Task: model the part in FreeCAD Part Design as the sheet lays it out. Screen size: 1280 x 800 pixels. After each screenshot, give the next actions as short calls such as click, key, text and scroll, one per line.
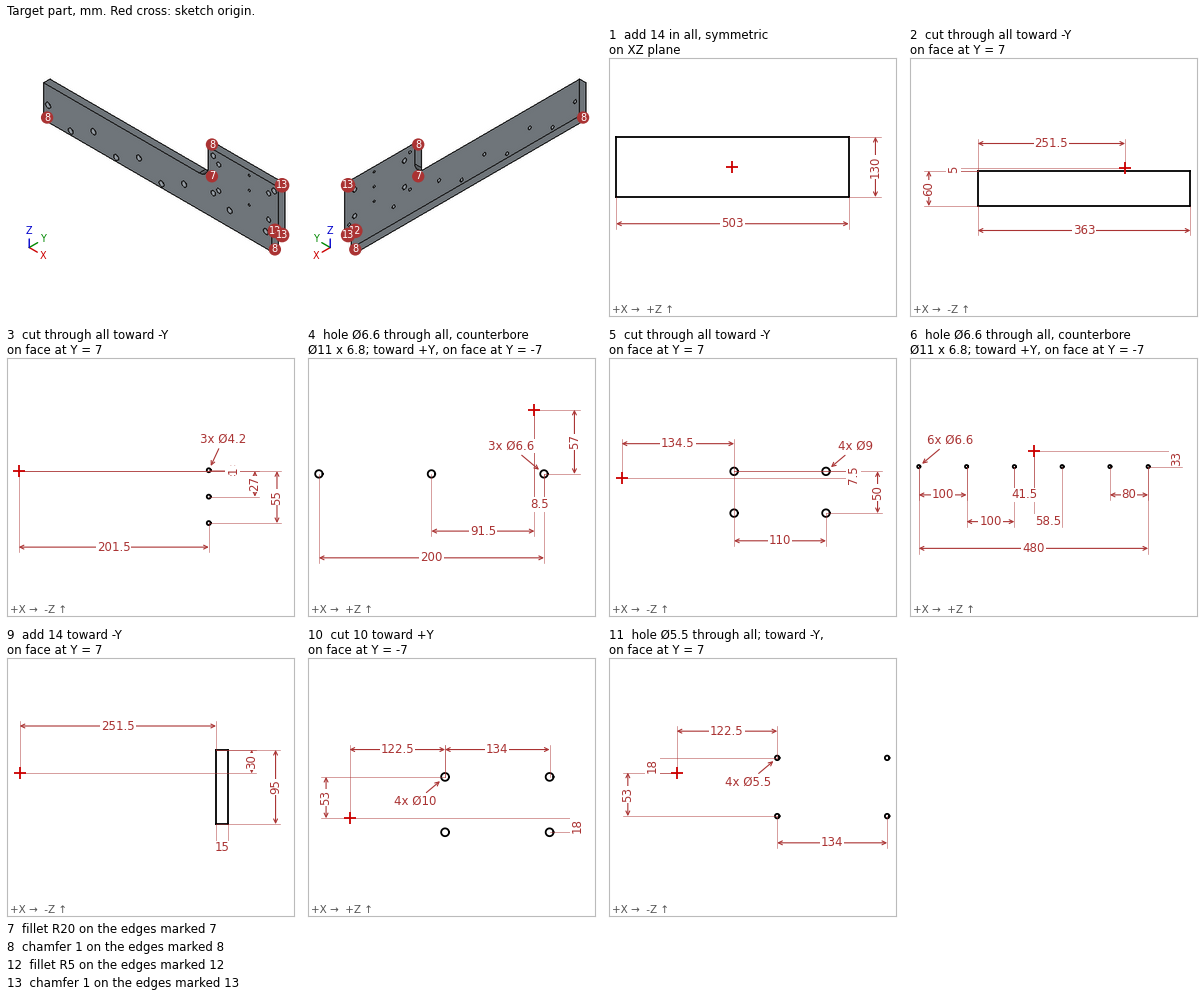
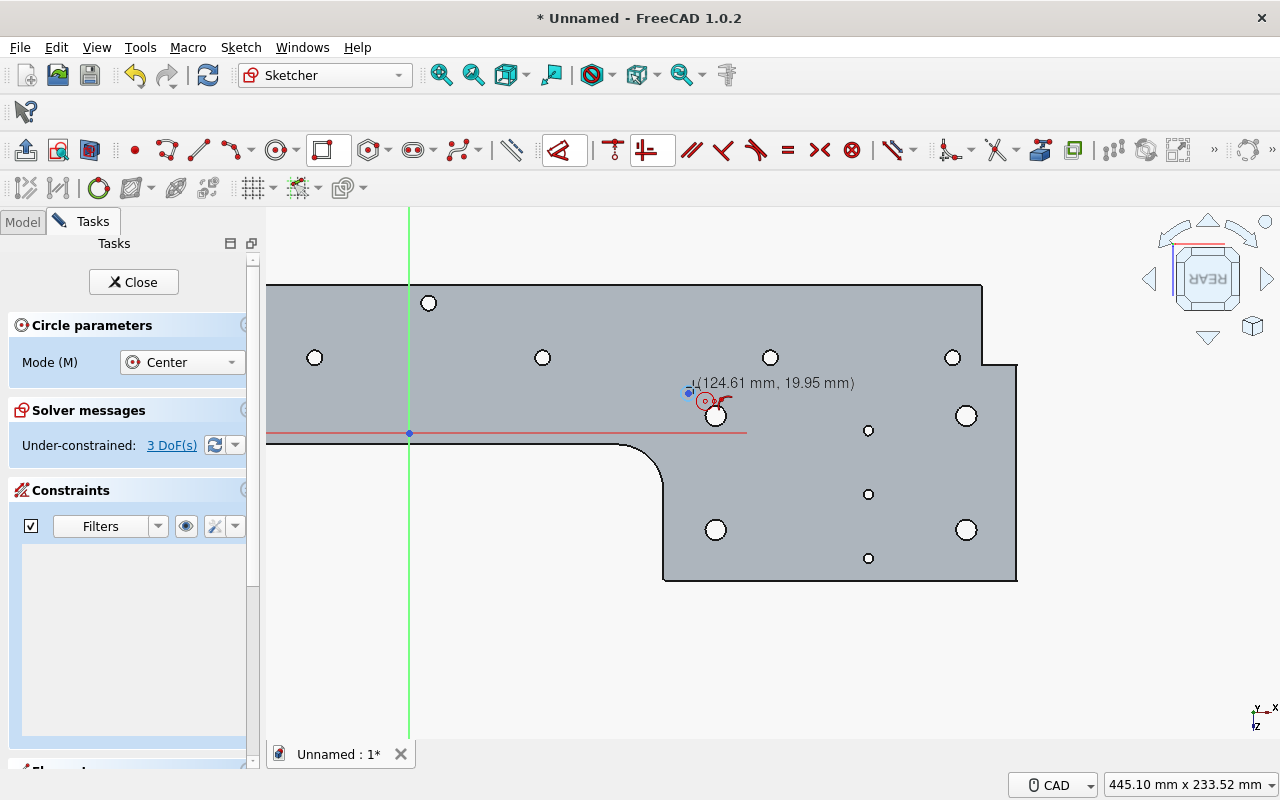
scroll(688, 554, up, 7)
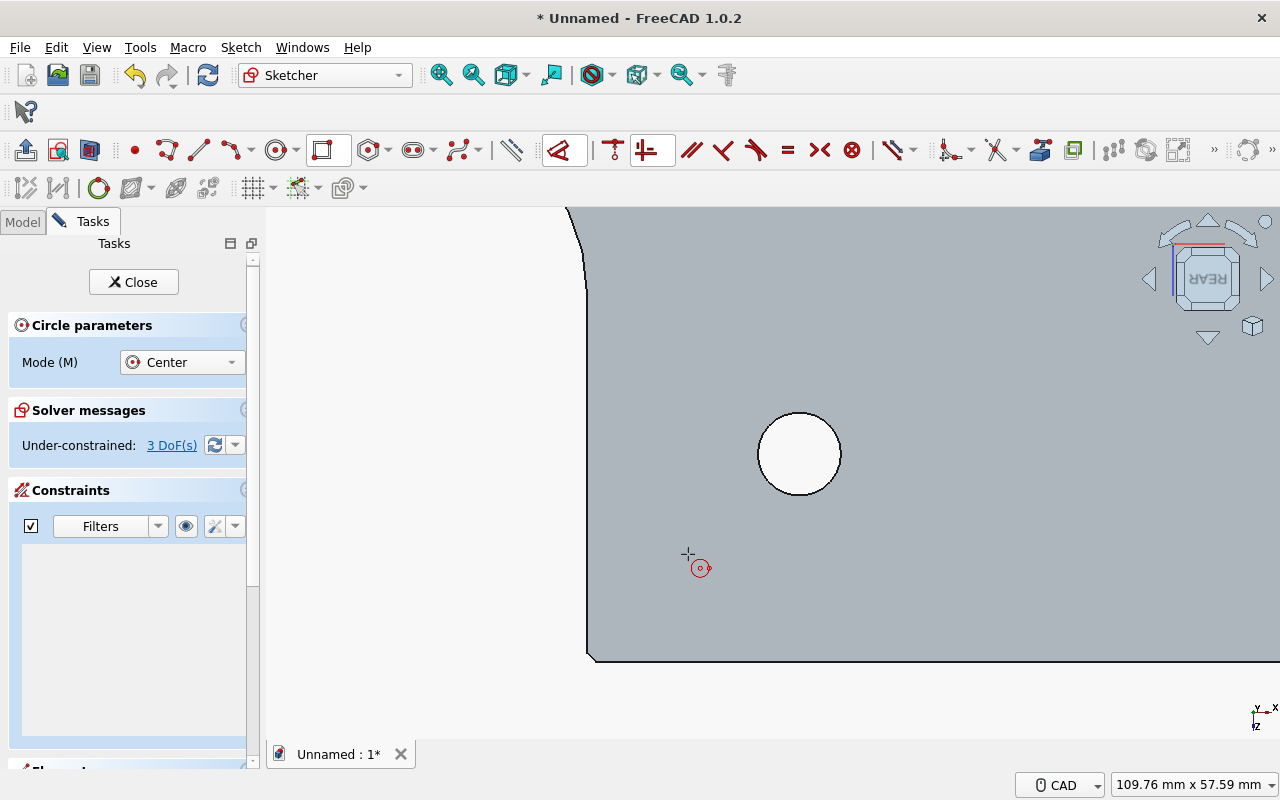
scroll(688, 555, down, 7)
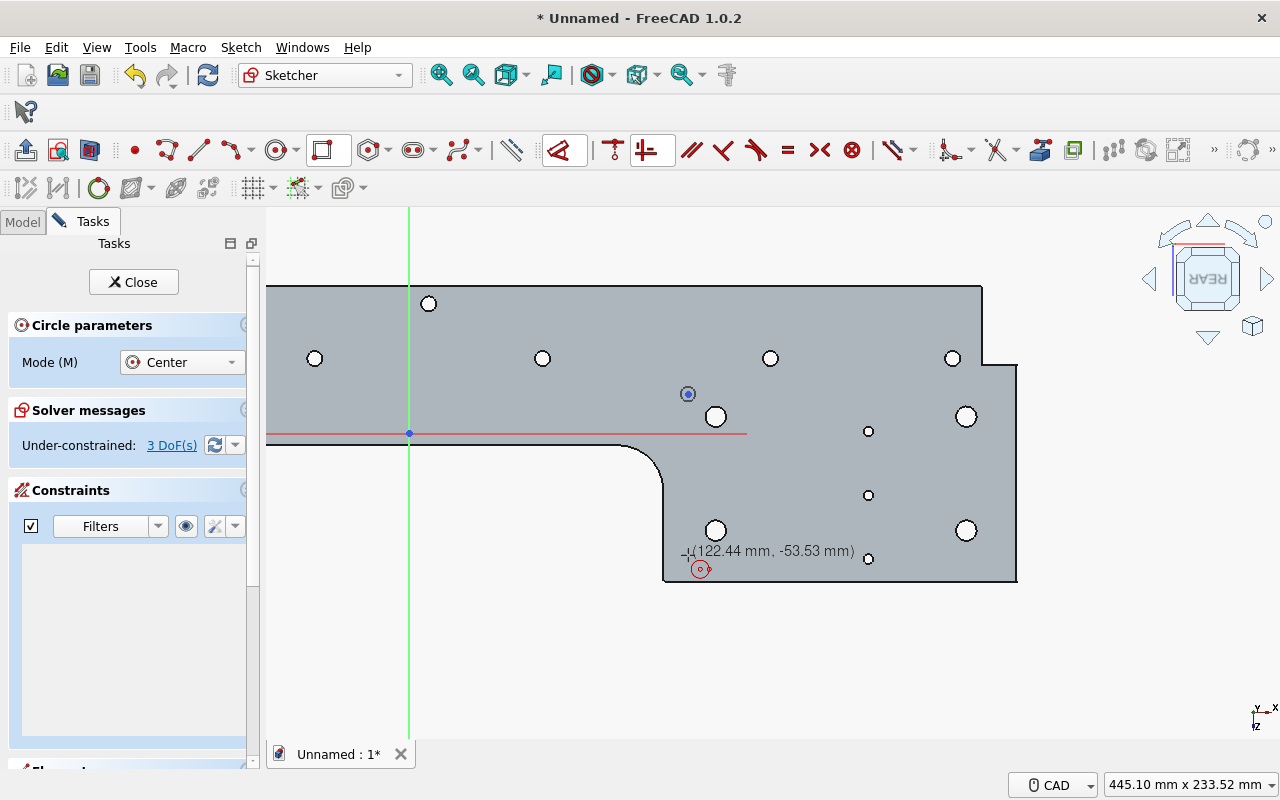
click(688, 555)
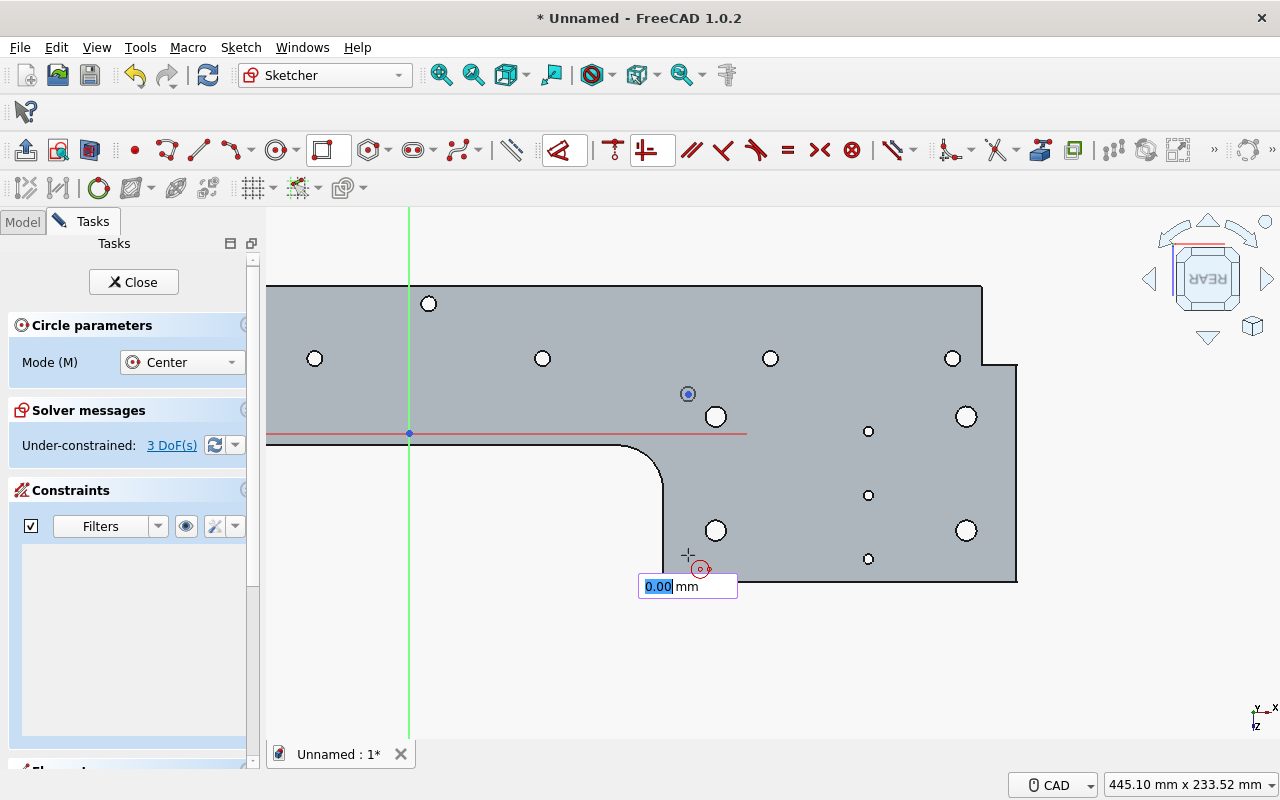
scroll(693, 550, up, 5)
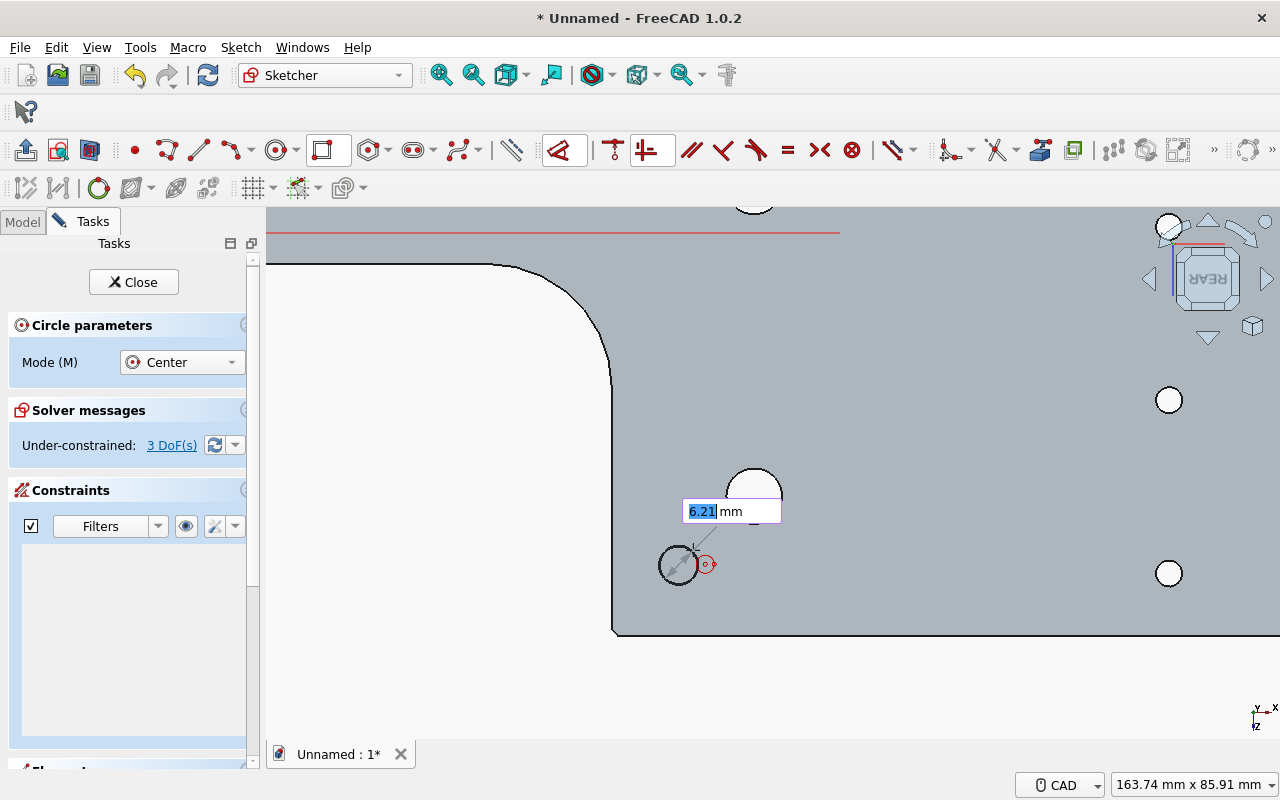
click(692, 549)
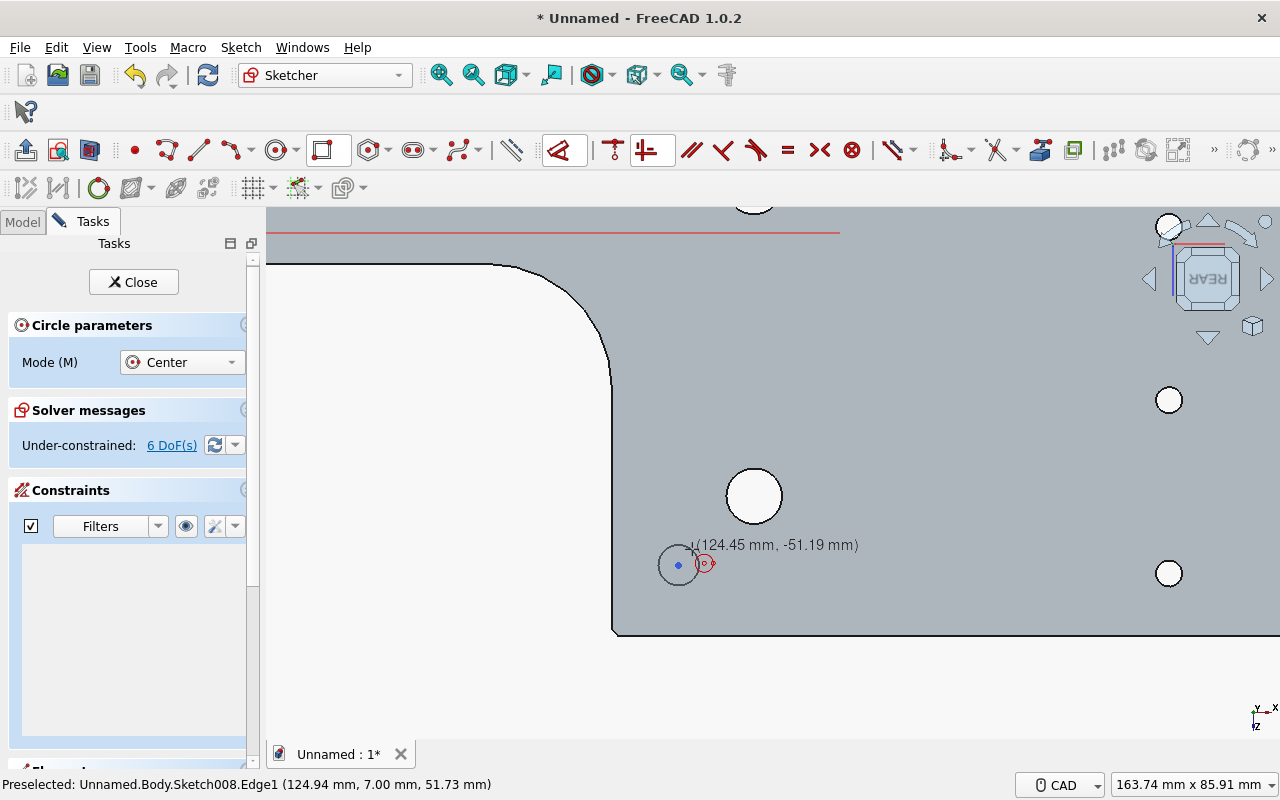
scroll(693, 550, down, 5)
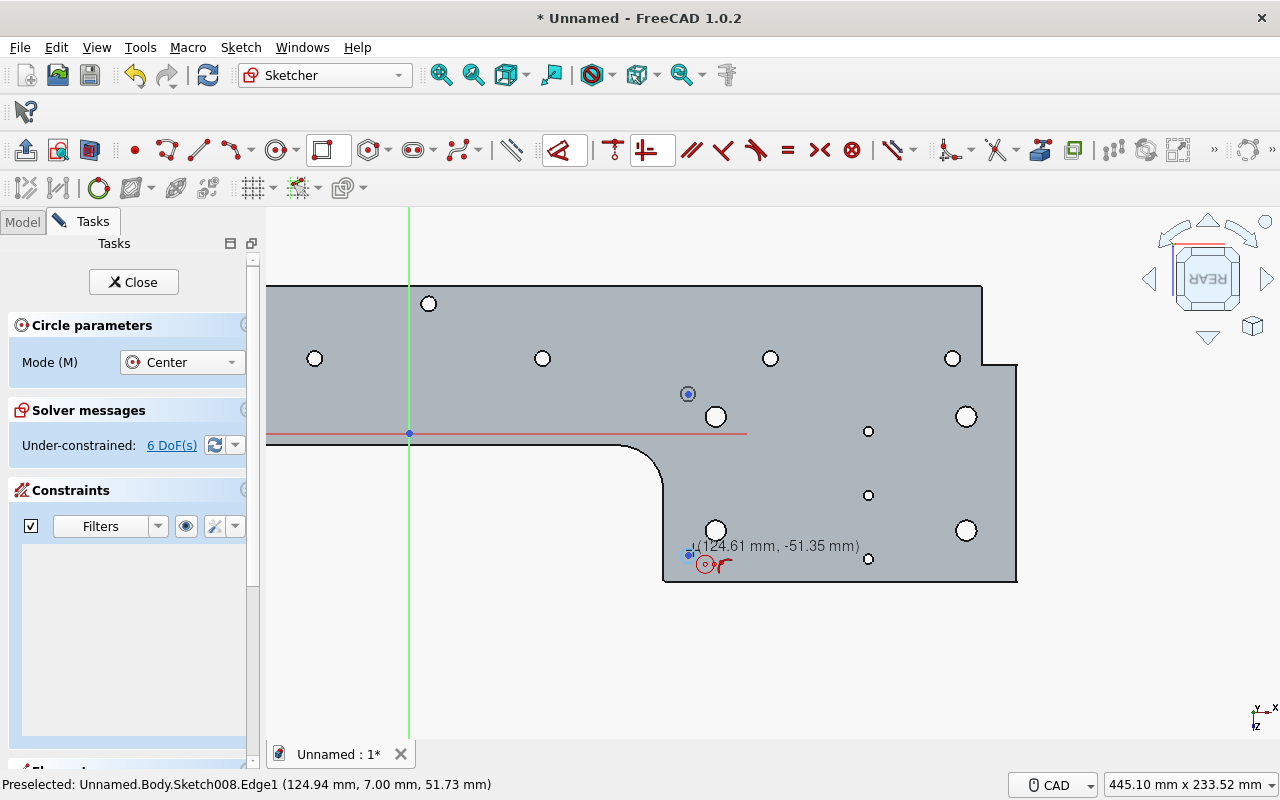
scroll(994, 555, up, 7)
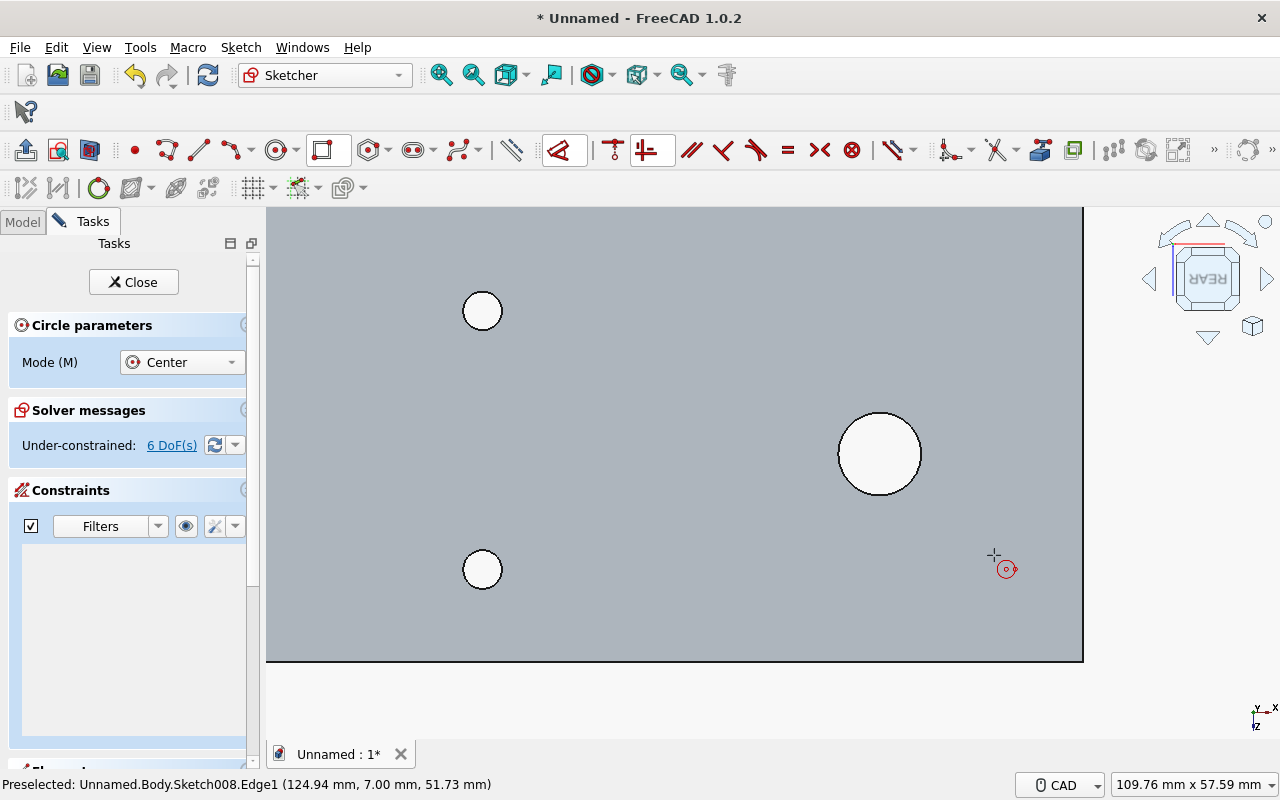
scroll(994, 555, down, 7)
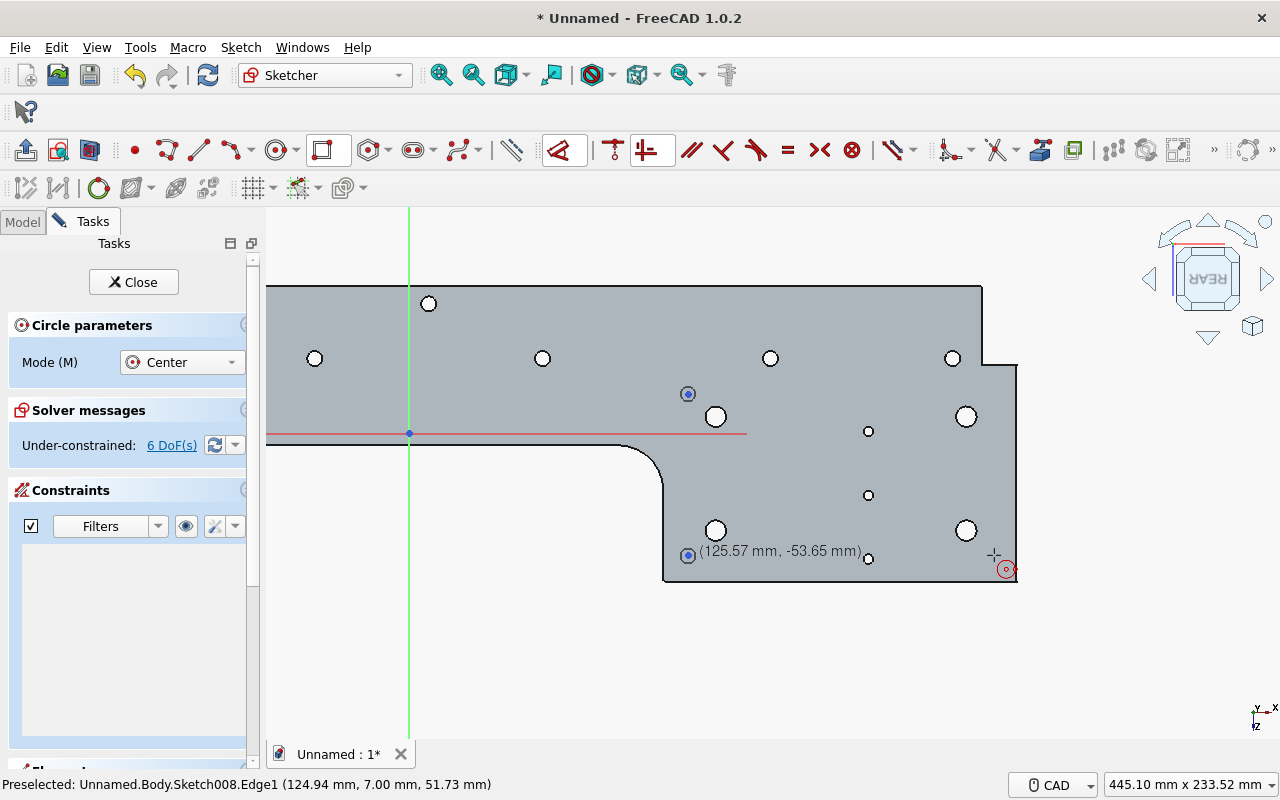
click(994, 555)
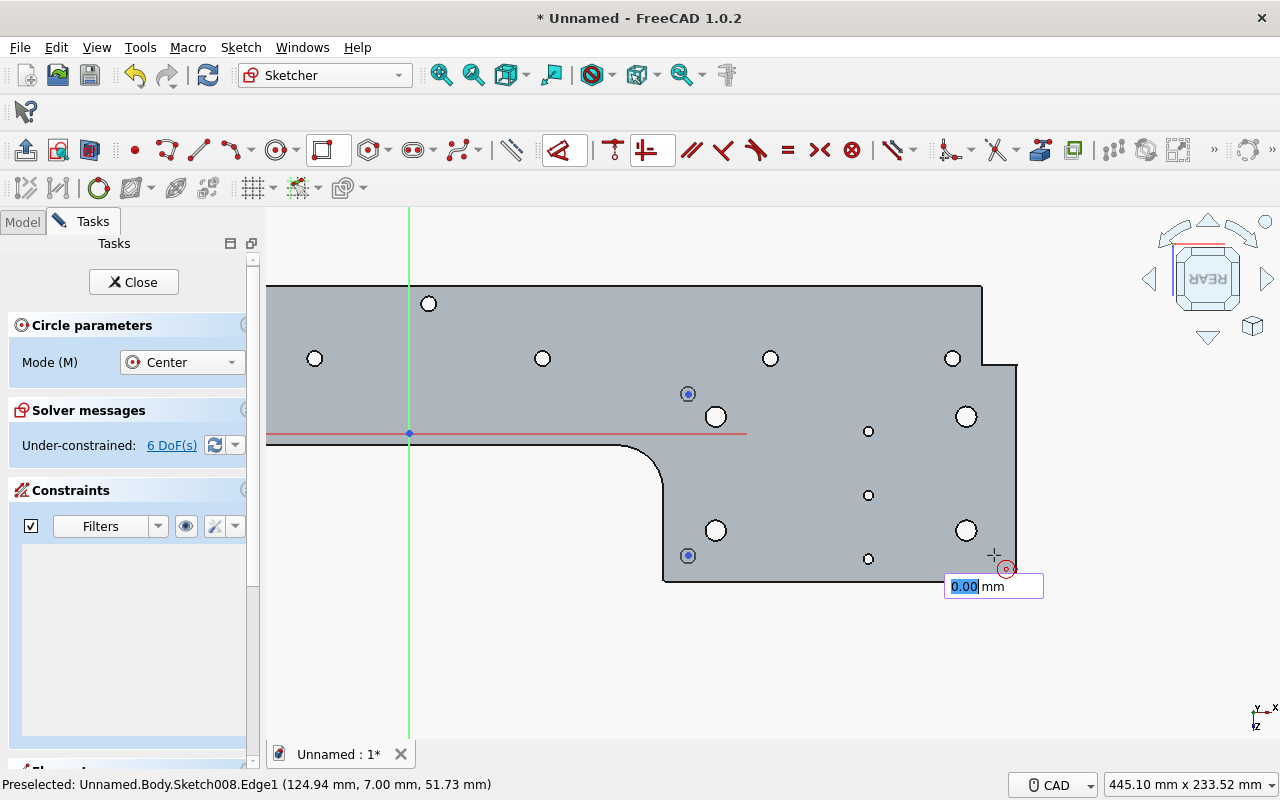
scroll(998, 550, up, 5)